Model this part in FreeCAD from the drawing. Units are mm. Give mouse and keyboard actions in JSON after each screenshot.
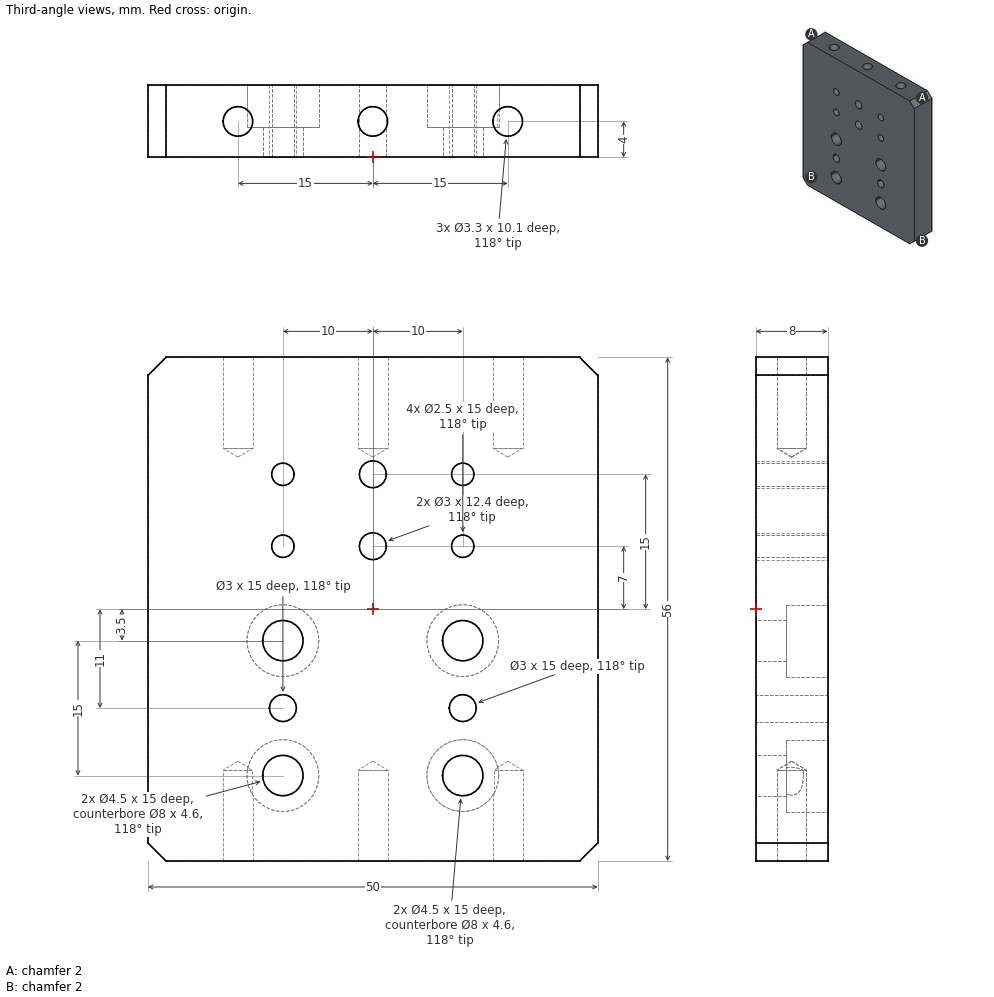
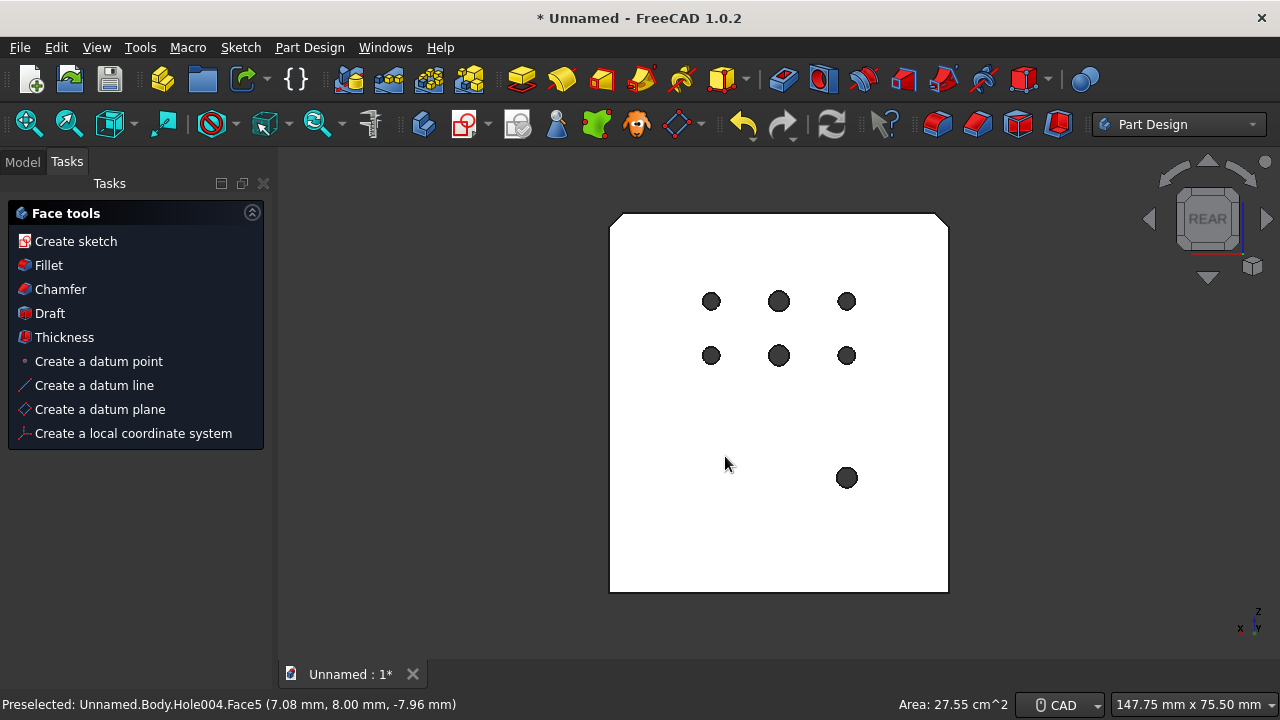
{"action": "left_click", "coordinate": [464, 124]}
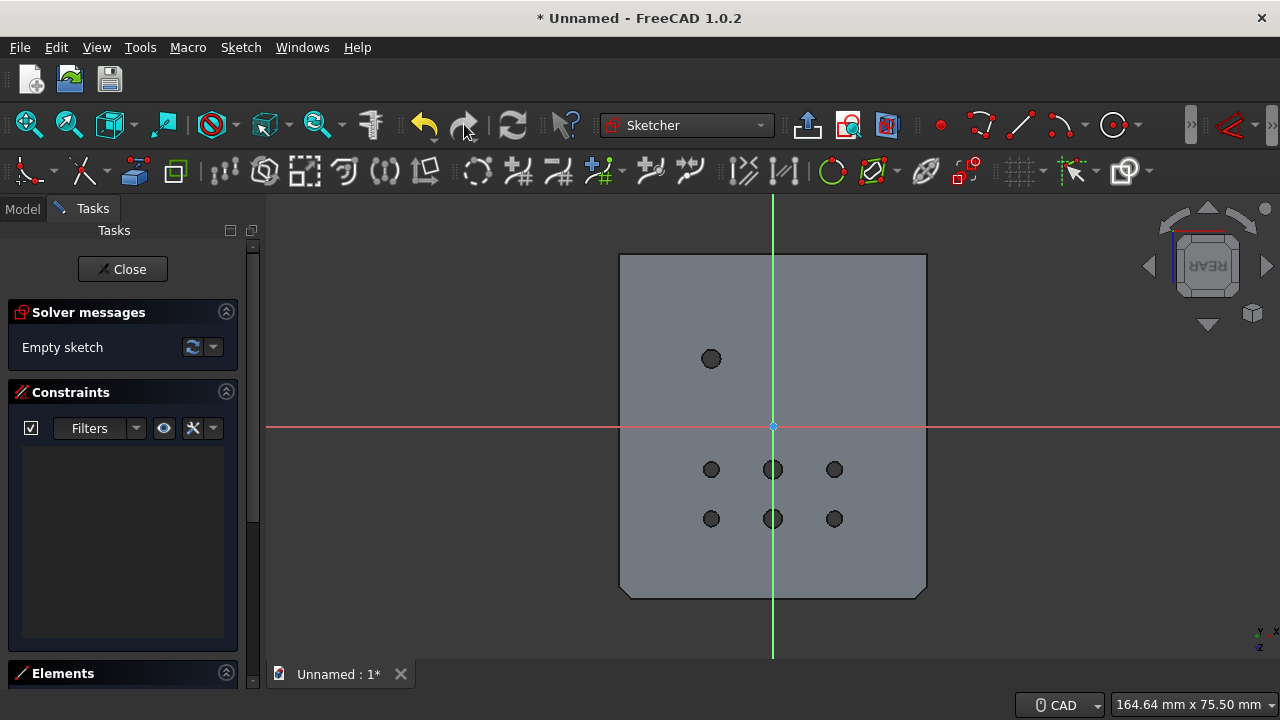
{"action": "scroll", "coordinate": [760, 310], "scroll_direction": "up", "scroll_amount": 4}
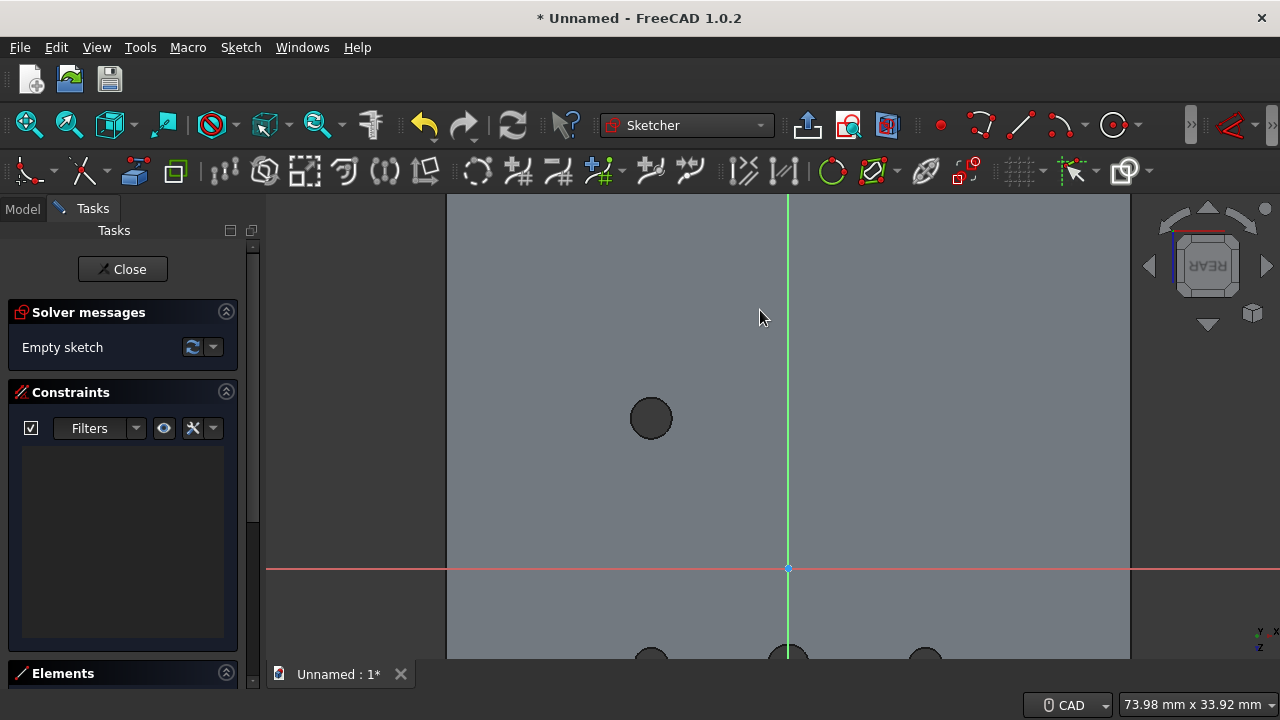
{"action": "left_click", "coordinate": [1114, 126]}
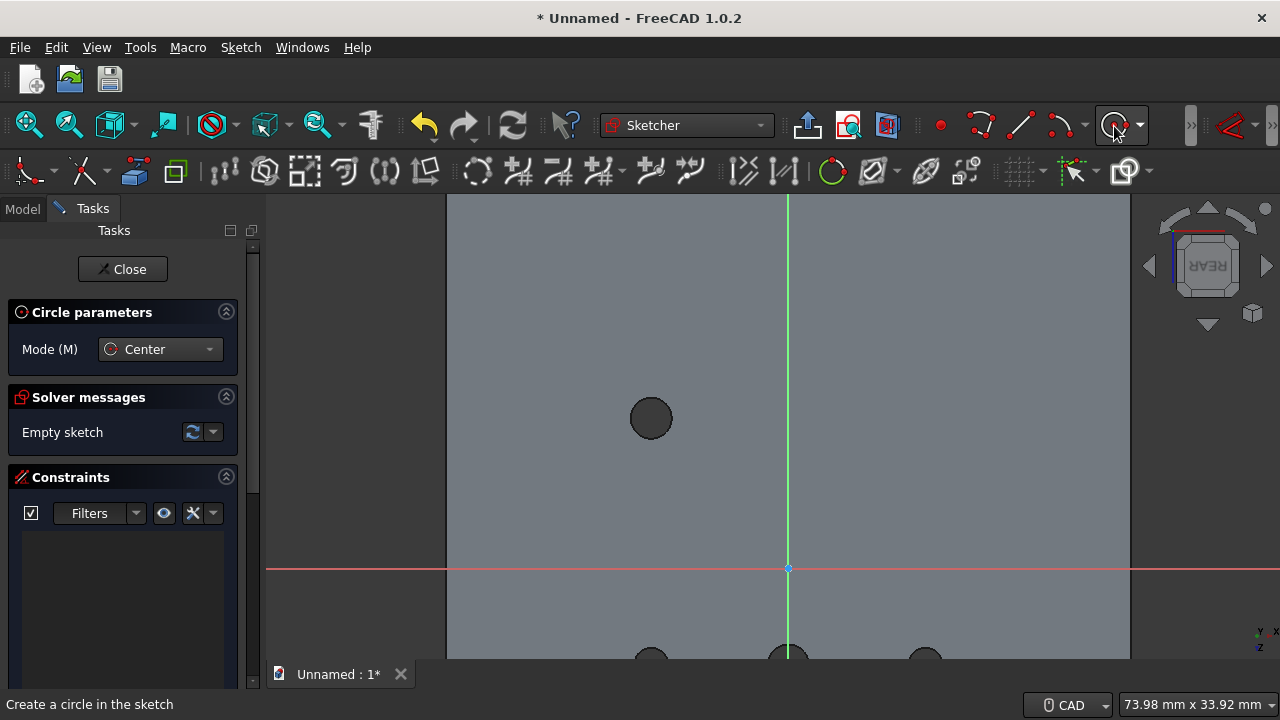
{"action": "left_click", "coordinate": [651, 315]}
{"action": "mouse_move", "coordinate": [673, 294]}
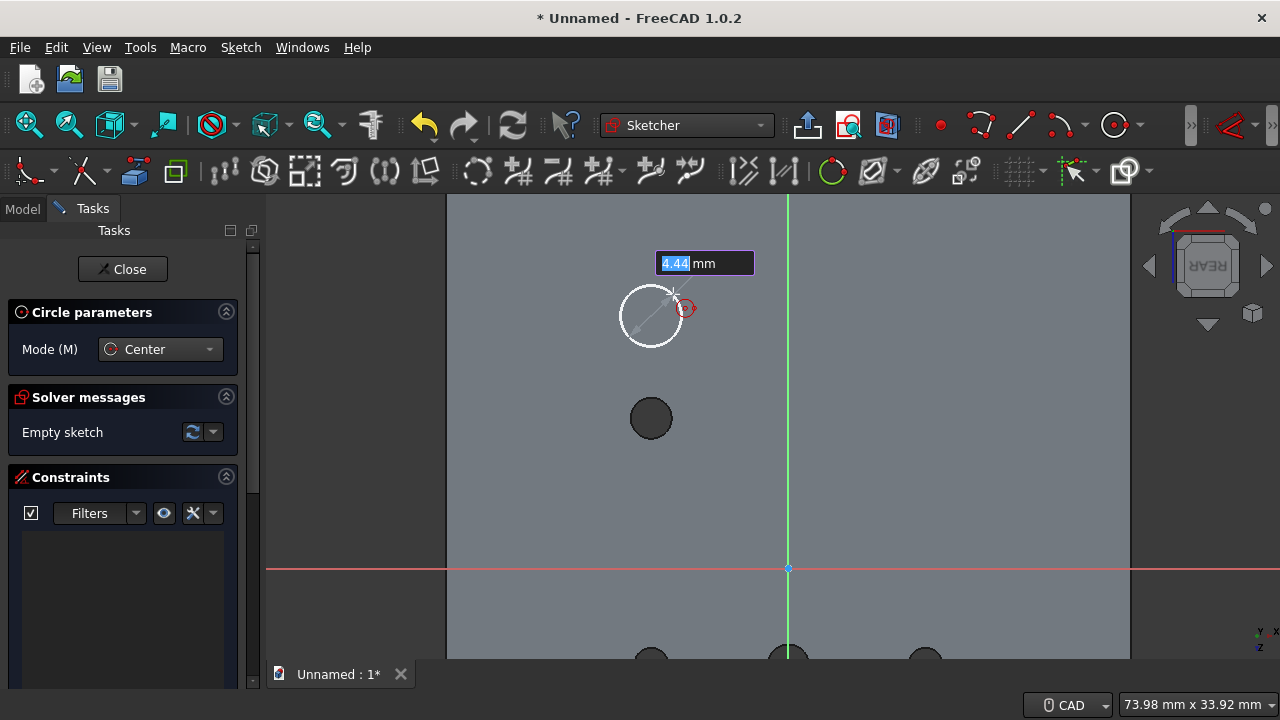
{"action": "type", "text": "4.5"}
{"action": "key", "text": "Return"}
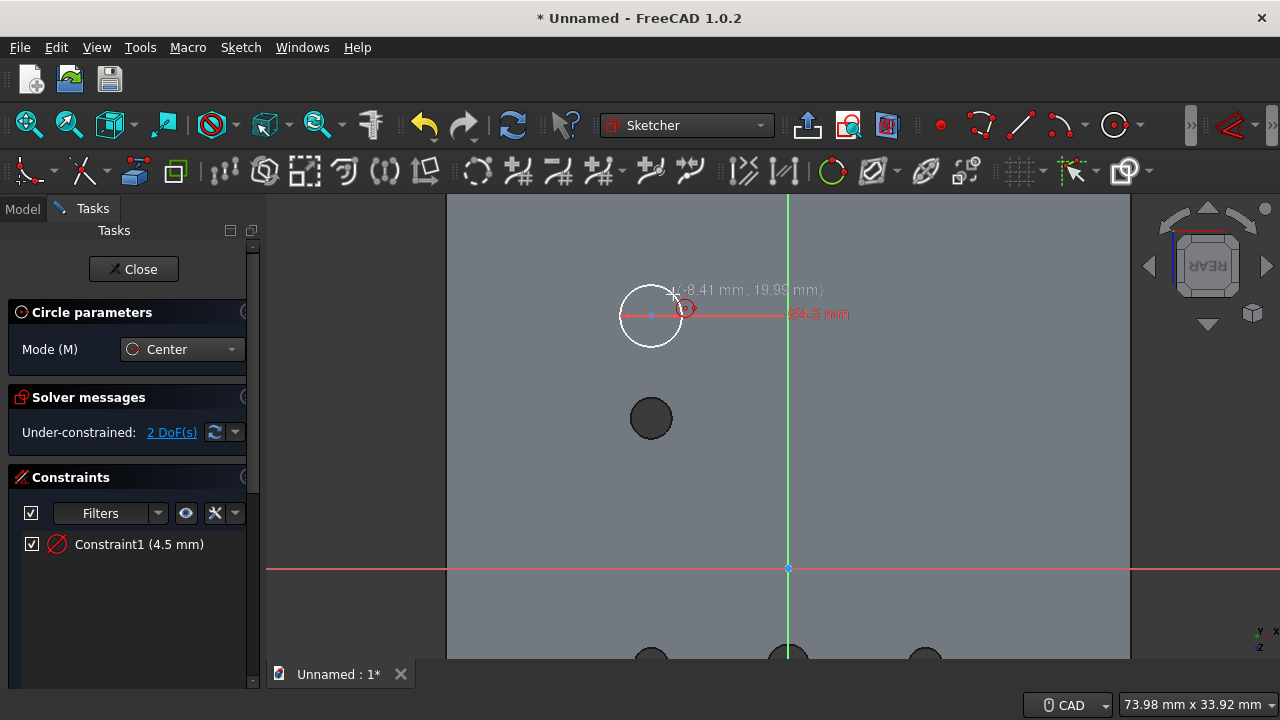
{"action": "left_click", "coordinate": [651, 521]}
{"action": "mouse_move", "coordinate": [673, 499]}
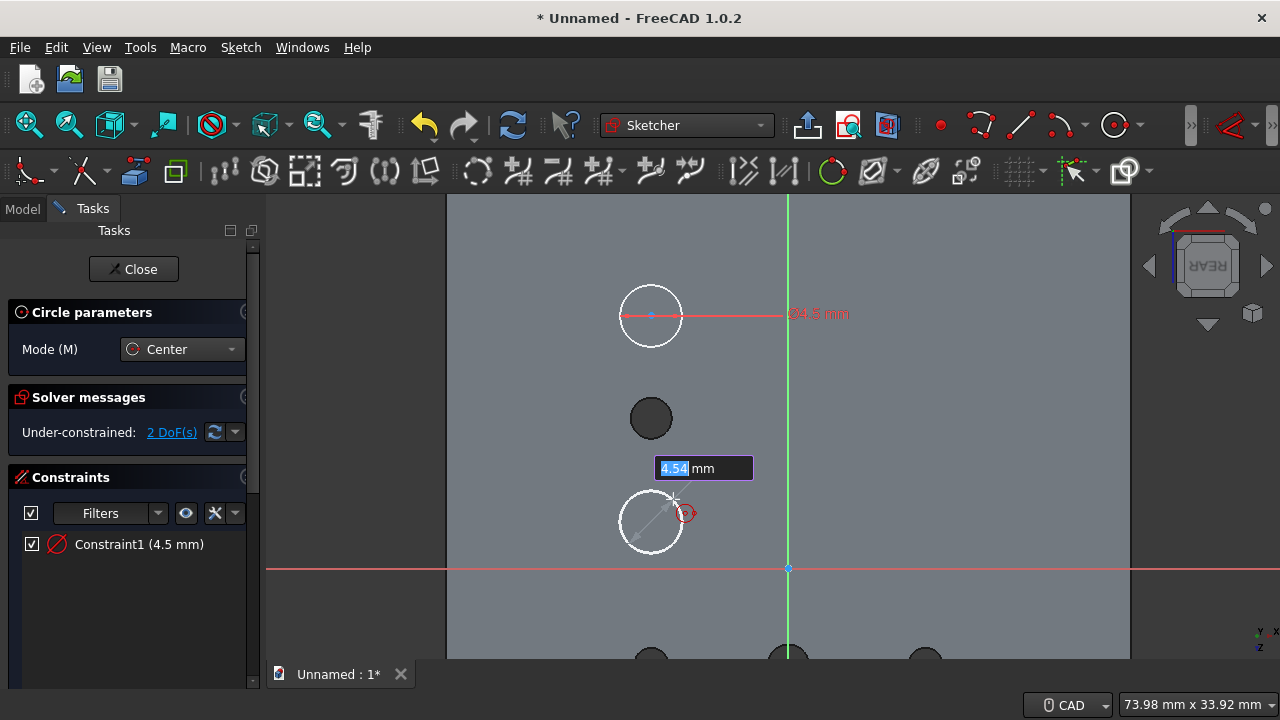
{"action": "type", "text": "4.5"}
{"action": "key", "text": "Return"}
{"action": "key", "text": "Escape"}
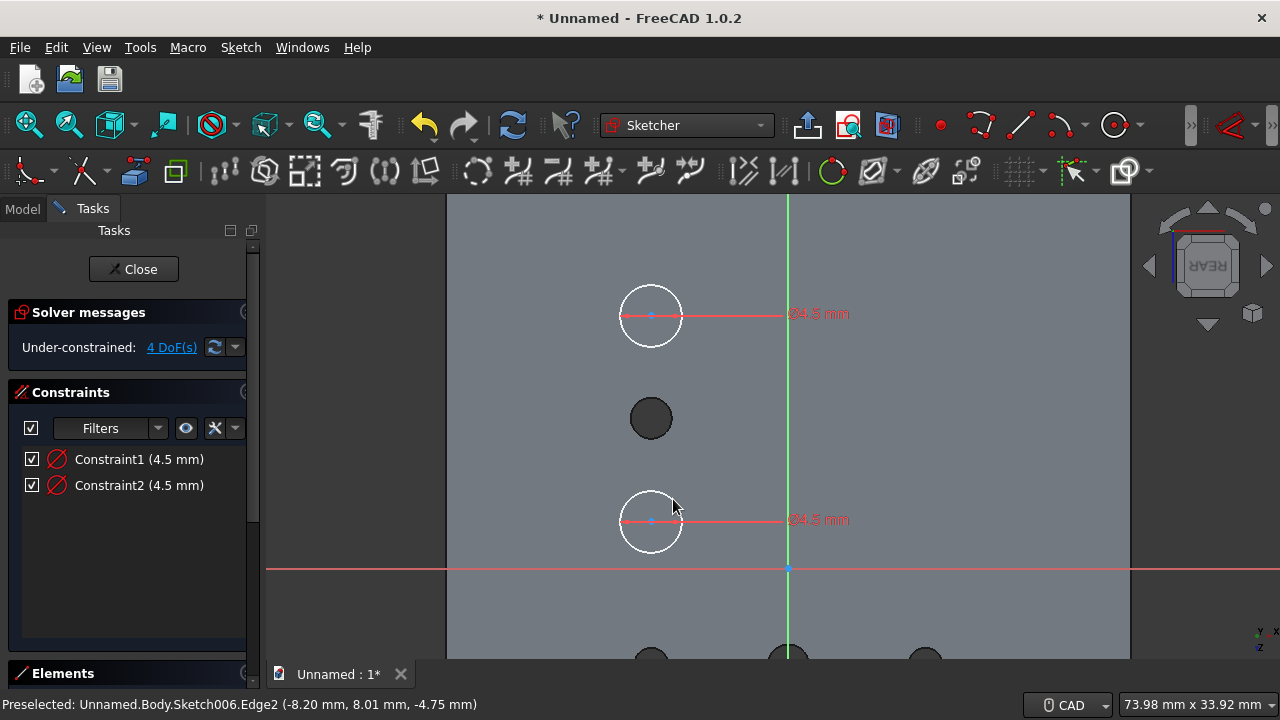
{"action": "left_click", "coordinate": [651, 316]}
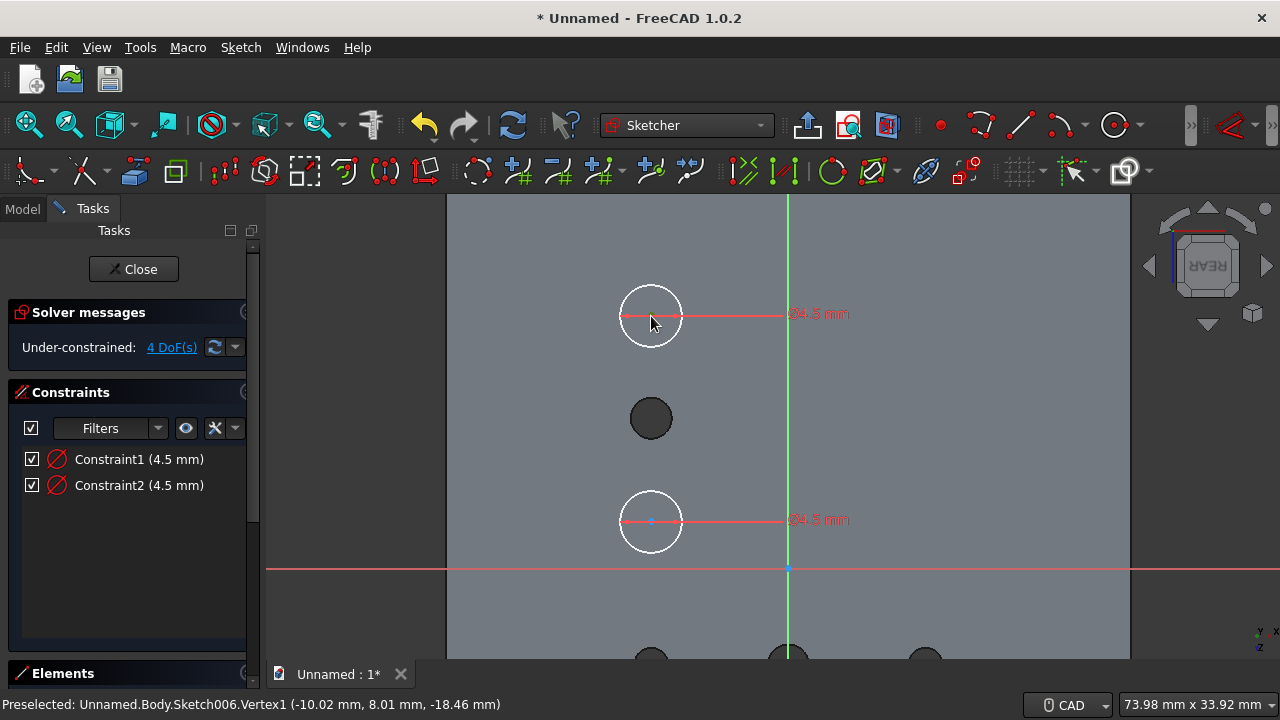
{"action": "left_click", "coordinate": [651, 522]}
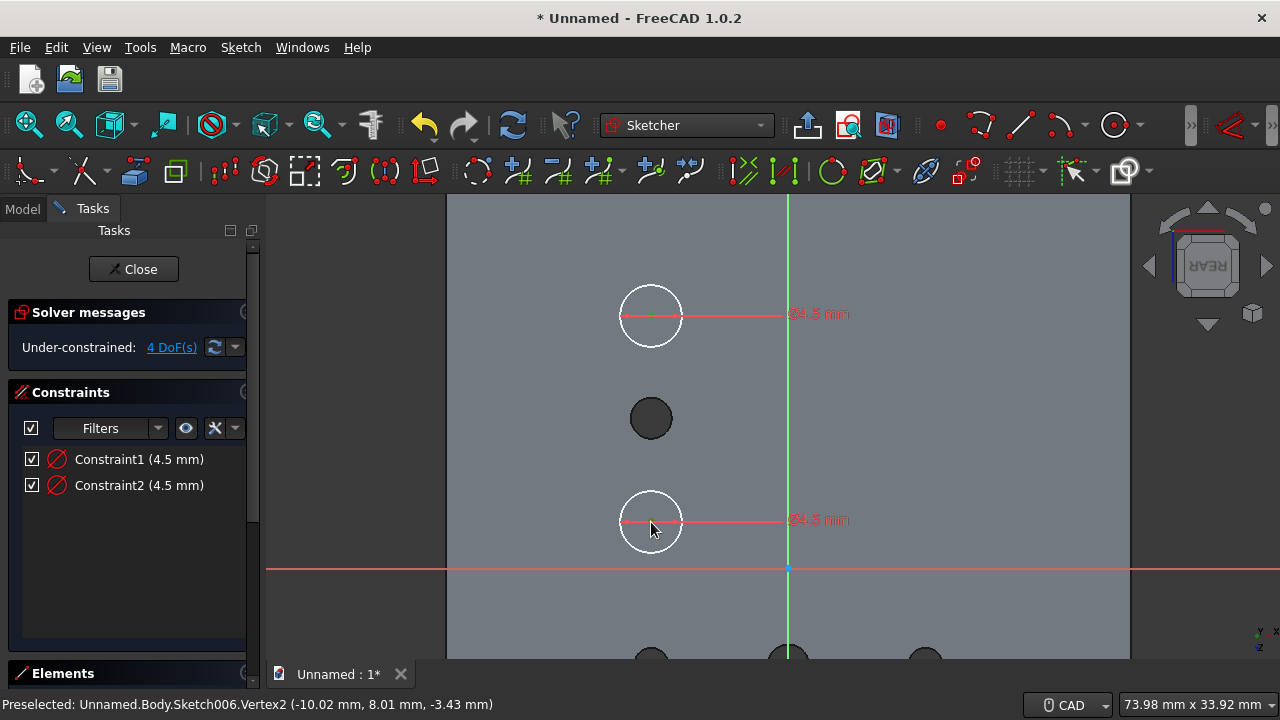
{"action": "key", "text": "v"}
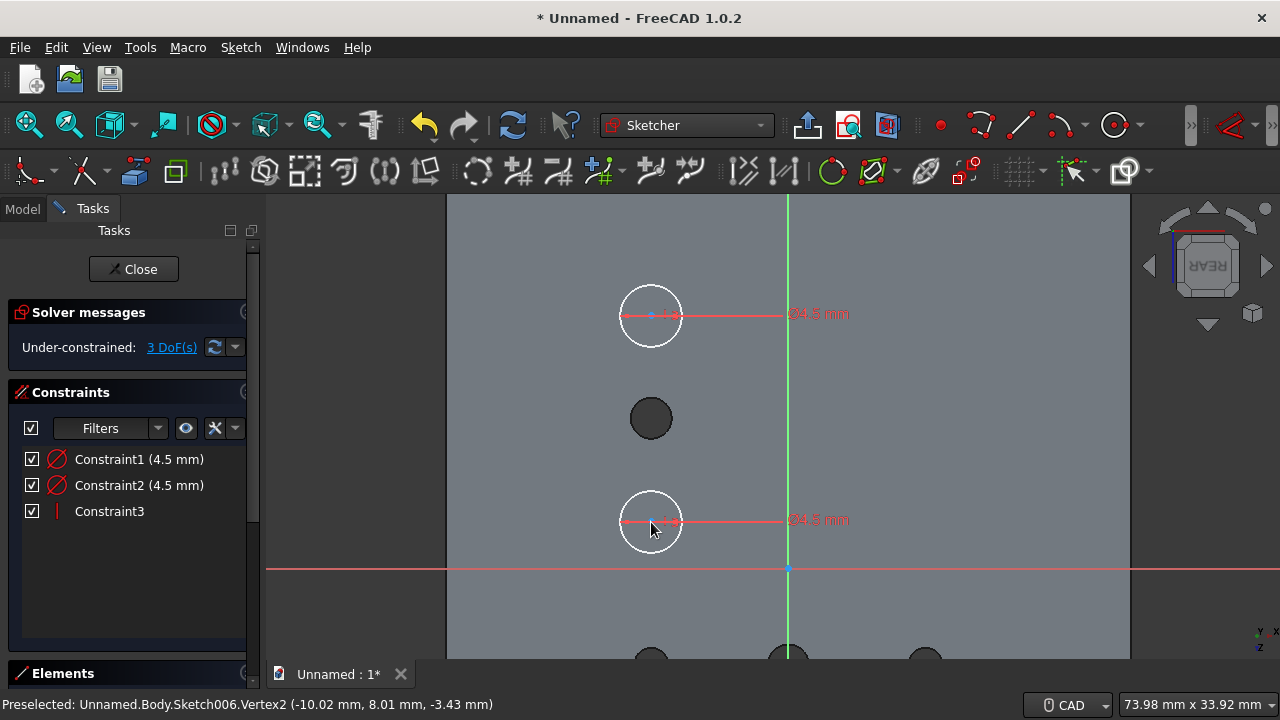
{"action": "left_click", "coordinate": [1230, 126]}